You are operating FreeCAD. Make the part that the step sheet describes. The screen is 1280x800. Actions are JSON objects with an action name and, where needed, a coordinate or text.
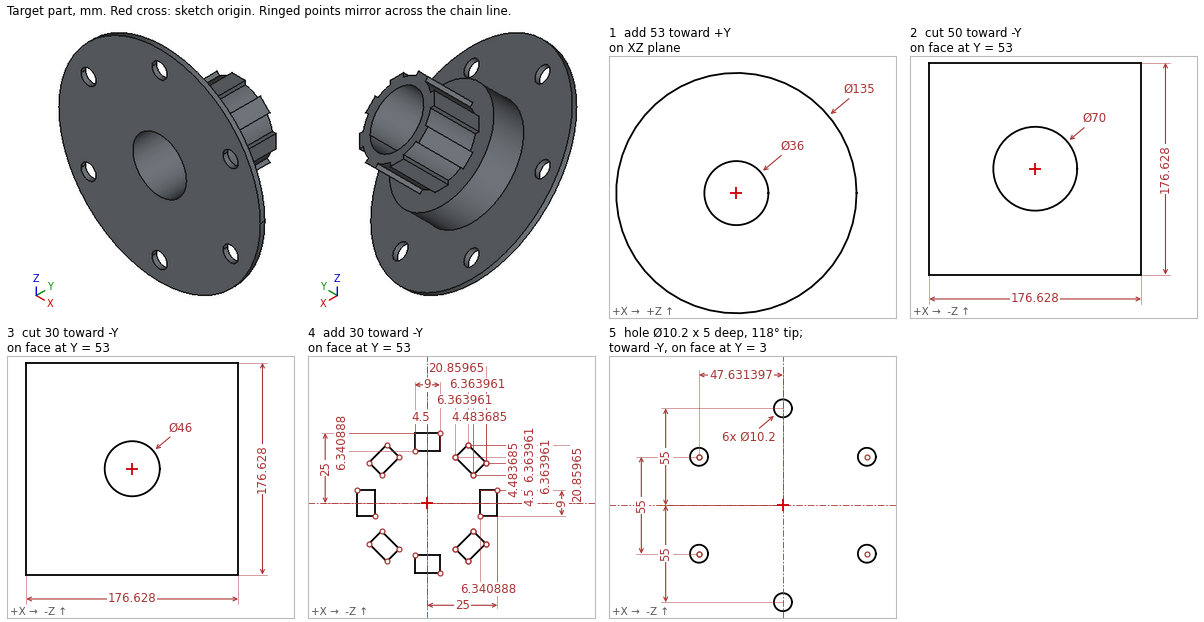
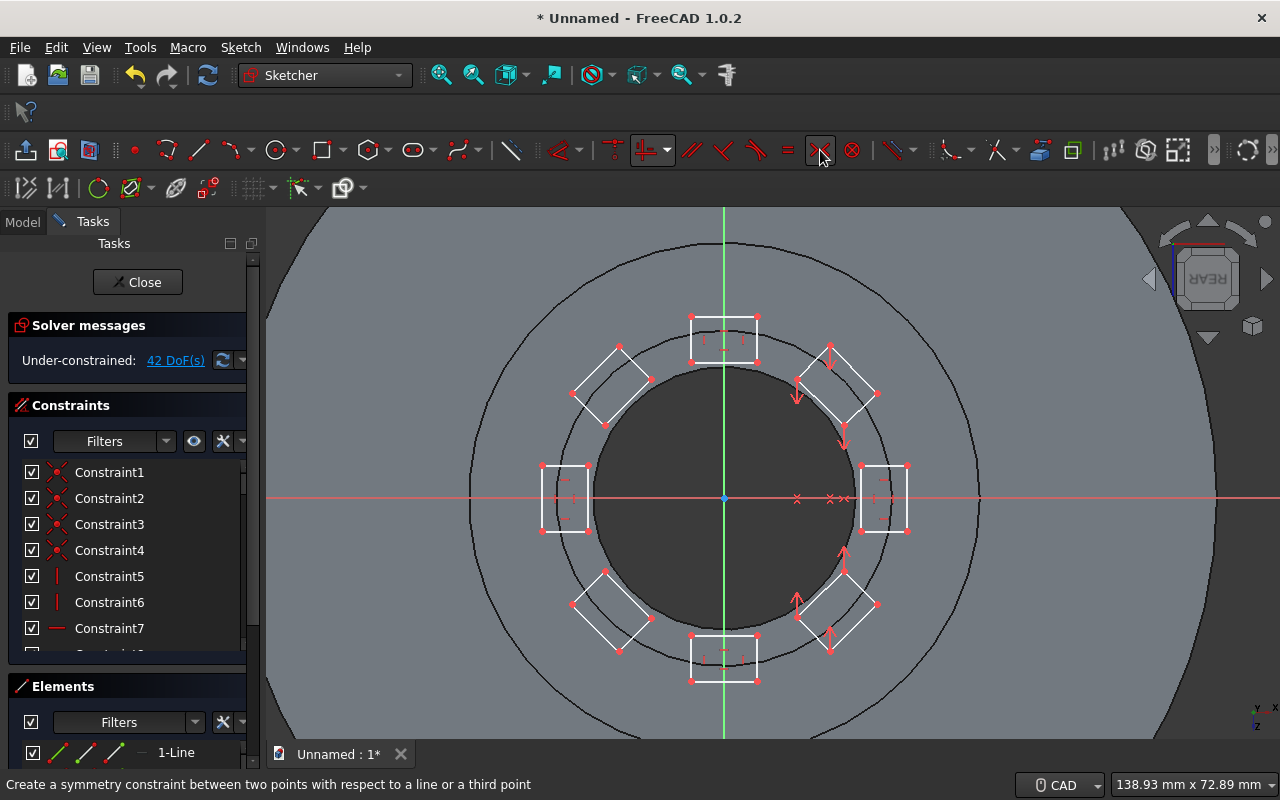
{"action": "left_click", "coordinate": [877, 394]}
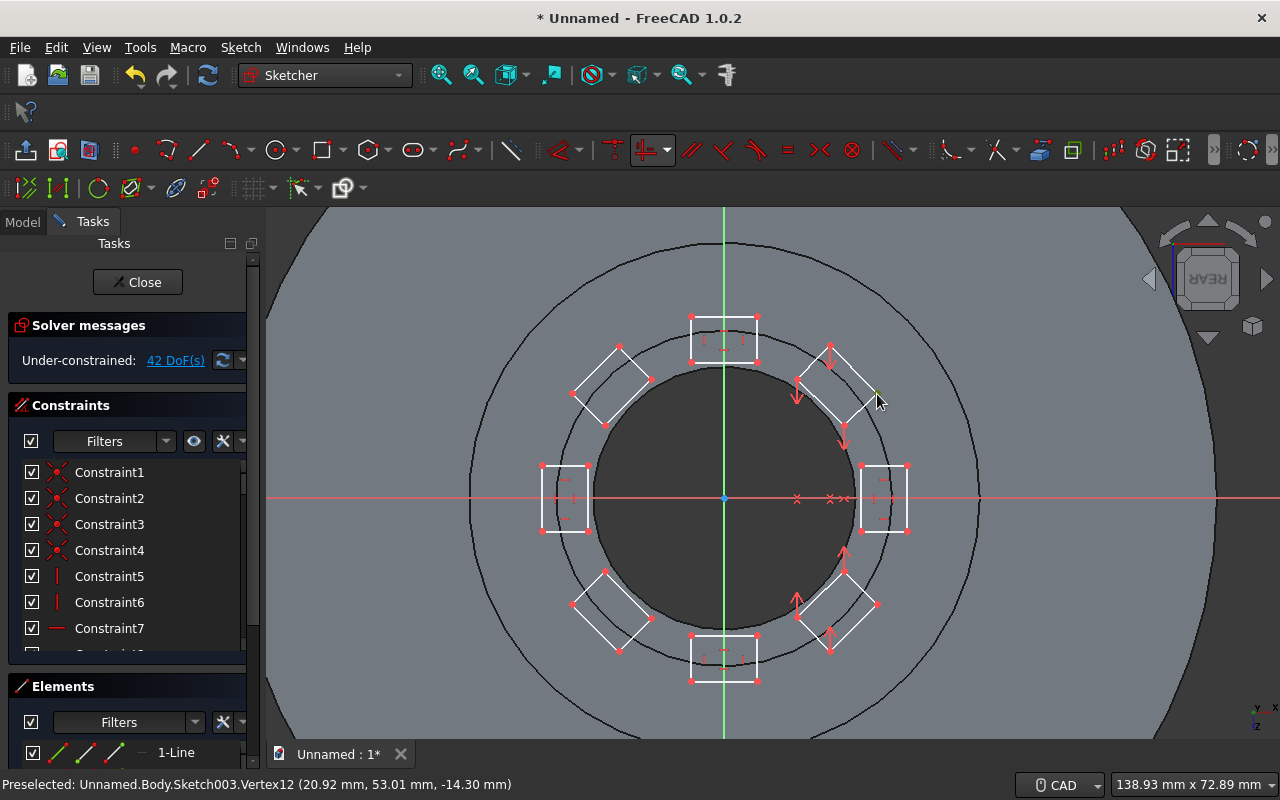
{"action": "left_click", "coordinate": [877, 605]}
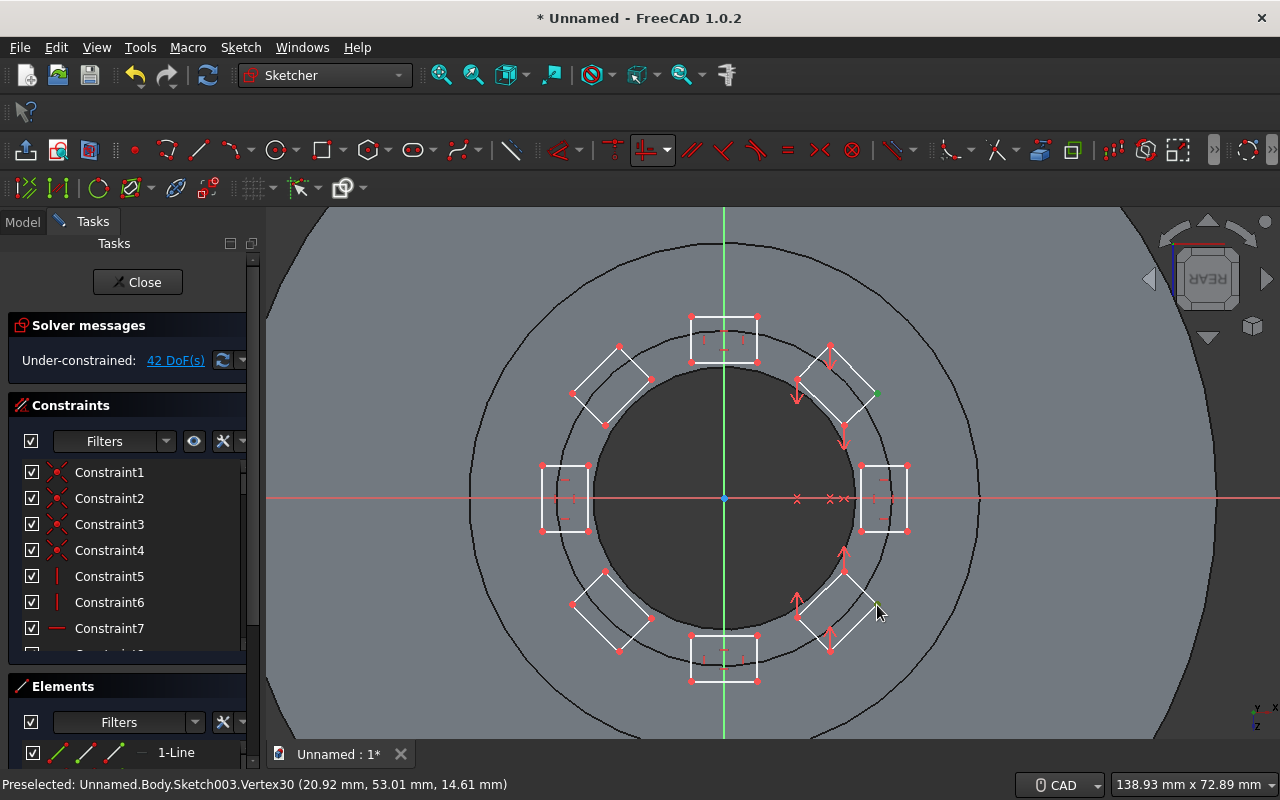
{"action": "left_click", "coordinate": [353, 498]}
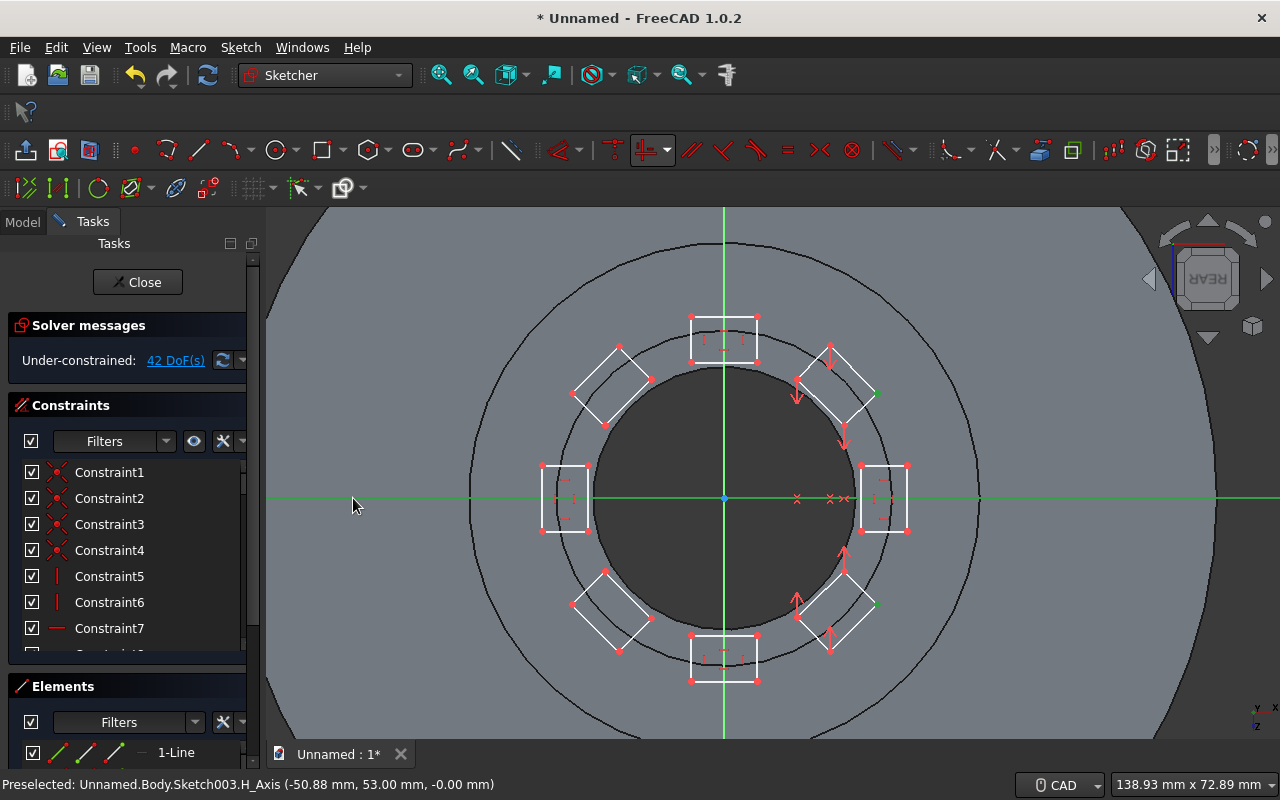
{"action": "left_click", "coordinate": [820, 150]}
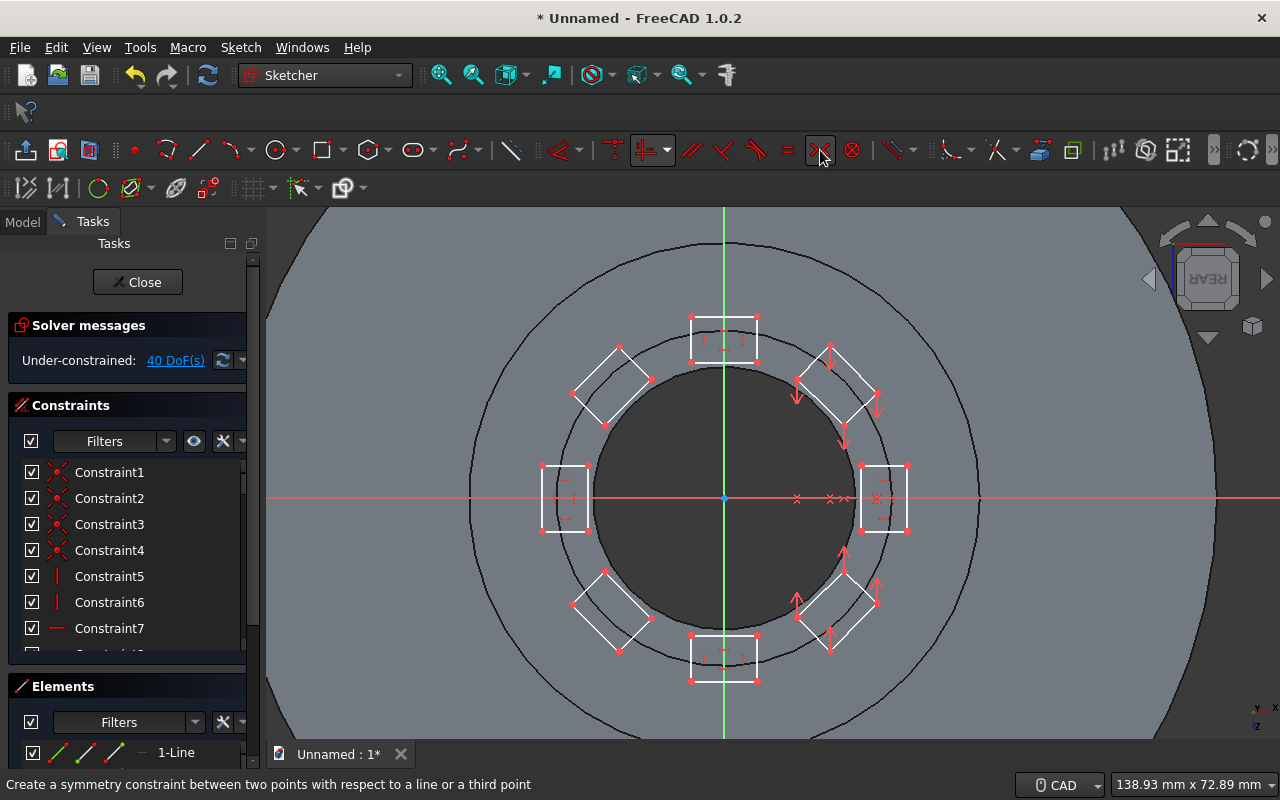
{"action": "left_click", "coordinate": [691, 363]}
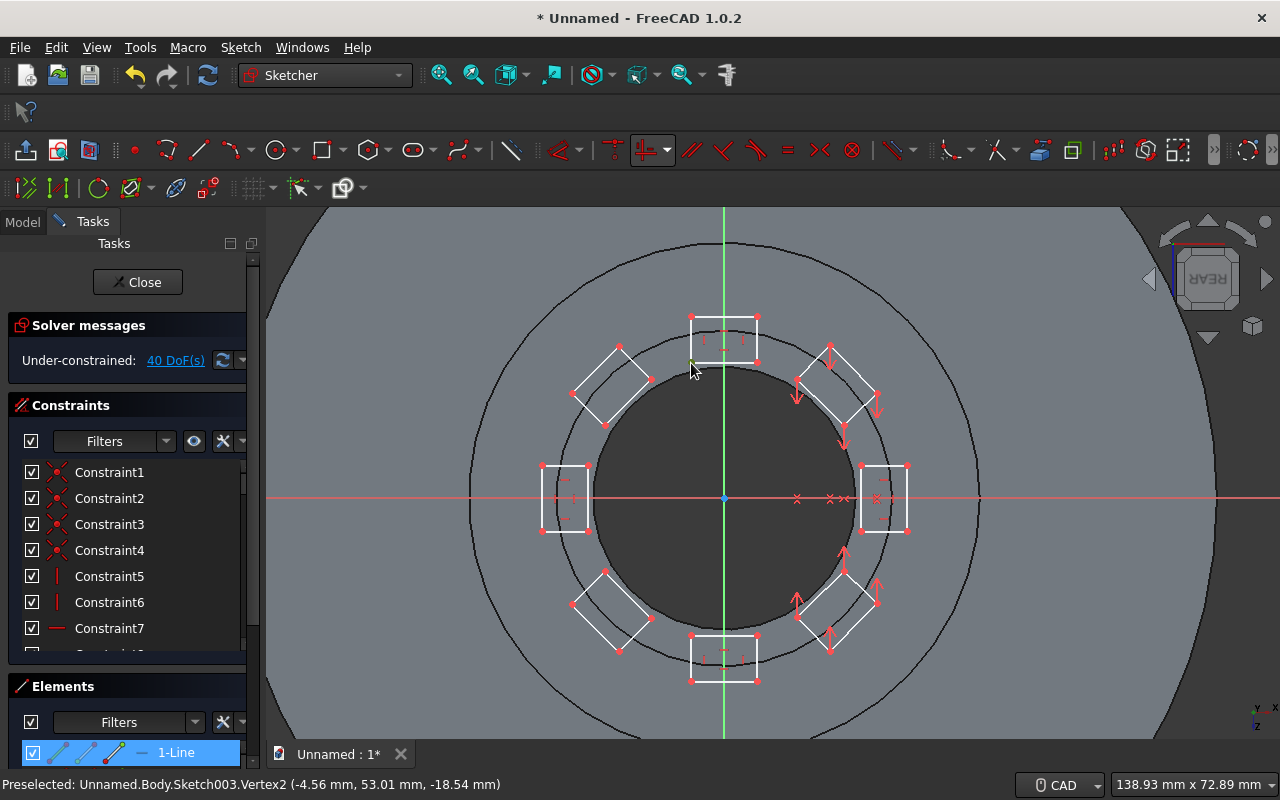
{"action": "left_click", "coordinate": [691, 636]}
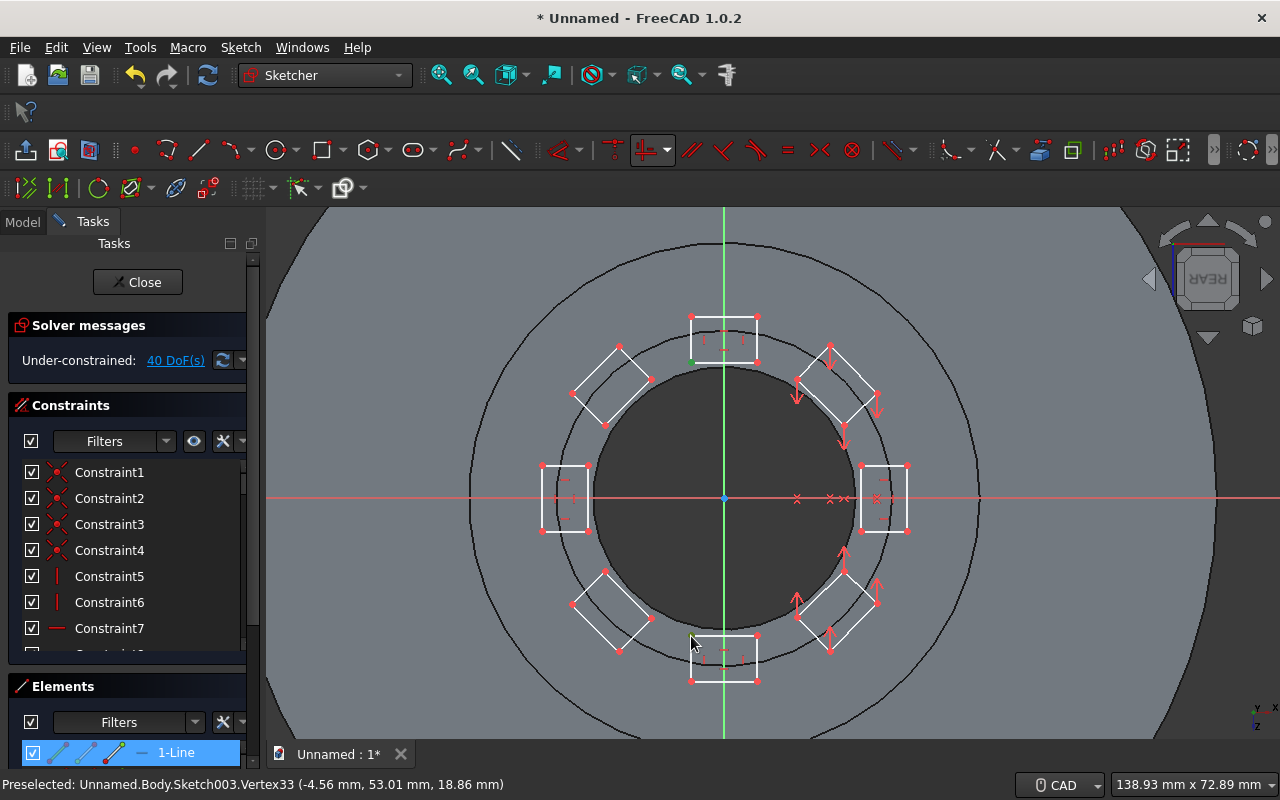
{"action": "left_click", "coordinate": [353, 498]}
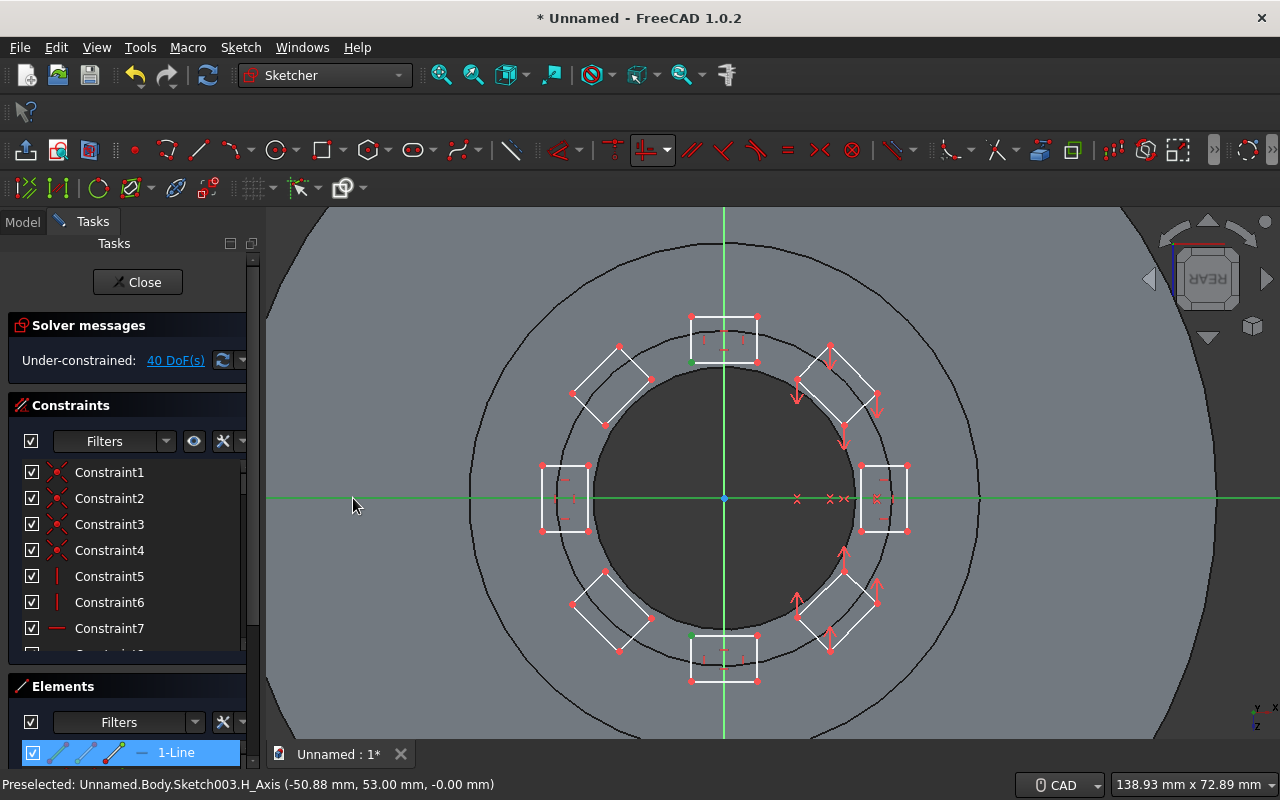
{"action": "left_click", "coordinate": [820, 150]}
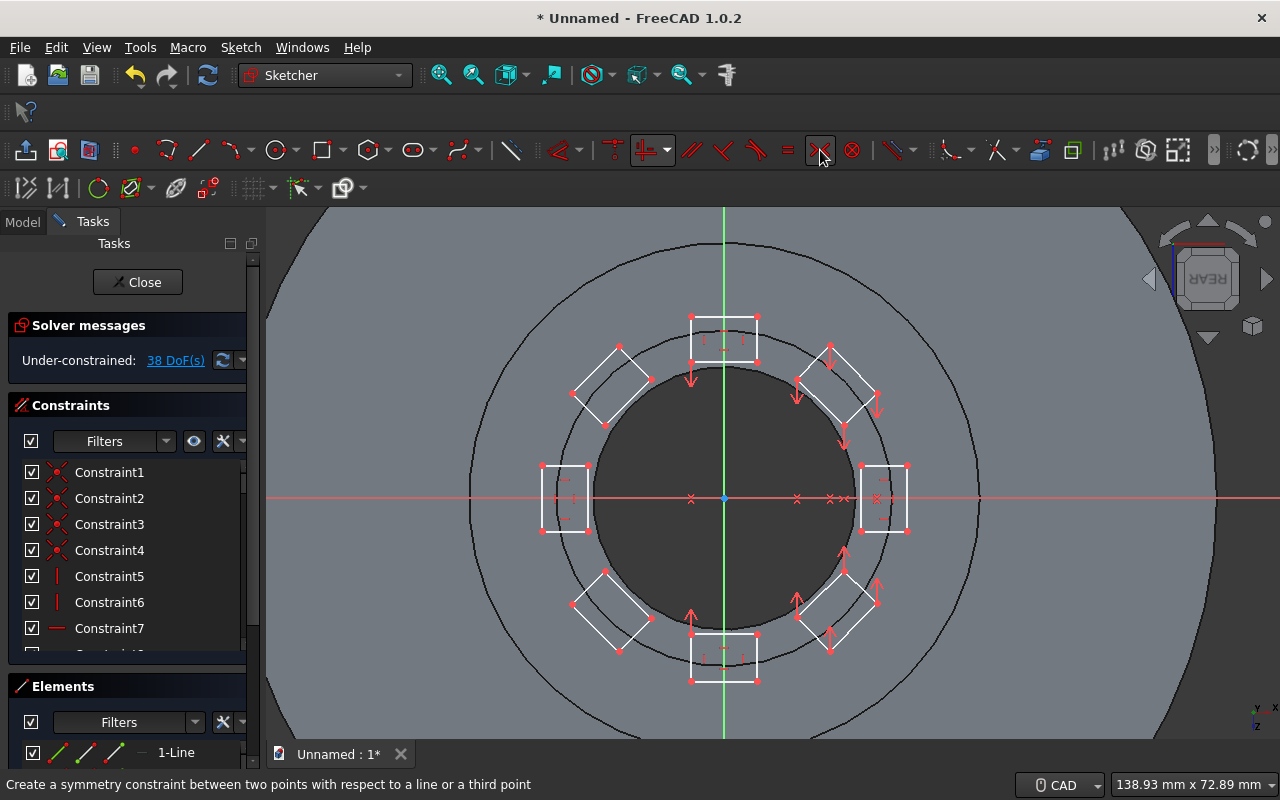
{"action": "left_click", "coordinate": [757, 317]}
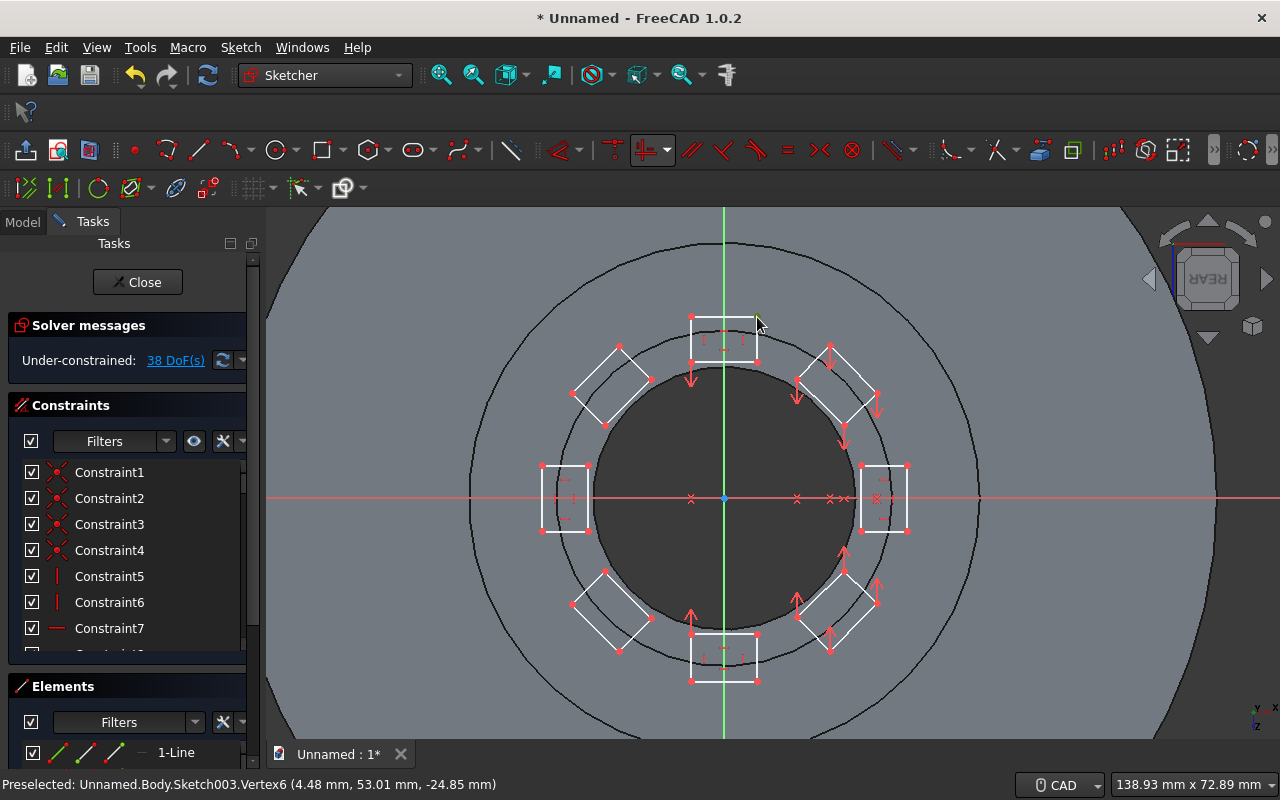
{"action": "left_click", "coordinate": [757, 682]}